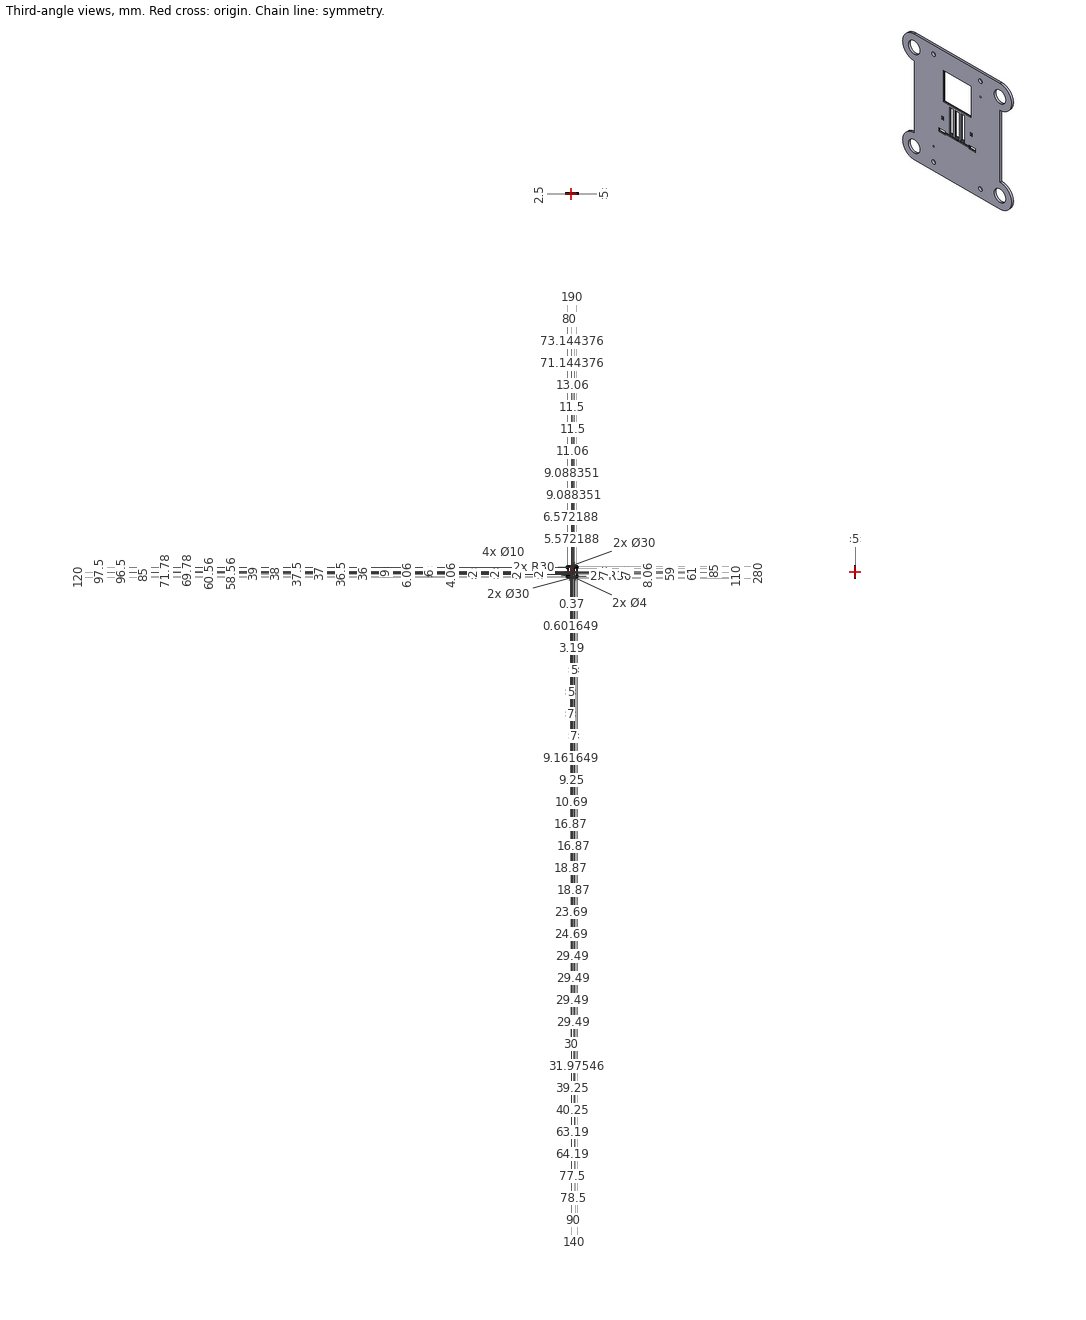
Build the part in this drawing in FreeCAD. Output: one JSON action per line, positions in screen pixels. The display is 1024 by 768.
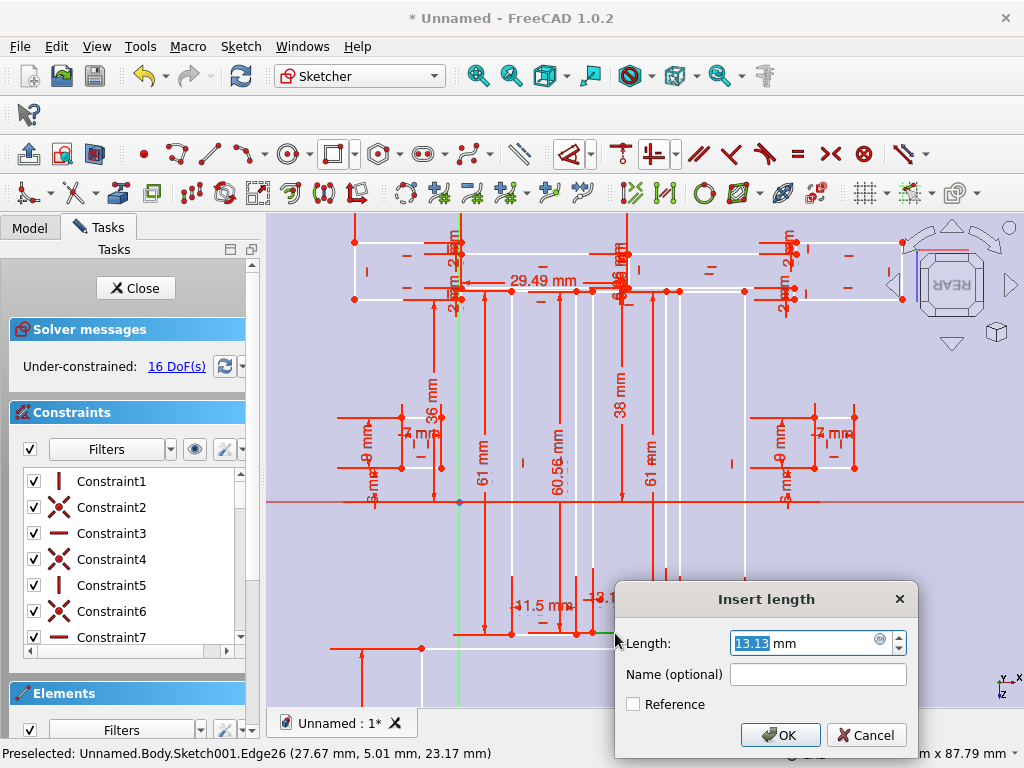
{"action": "type", "text": "13.06"}
{"action": "key", "text": "Return"}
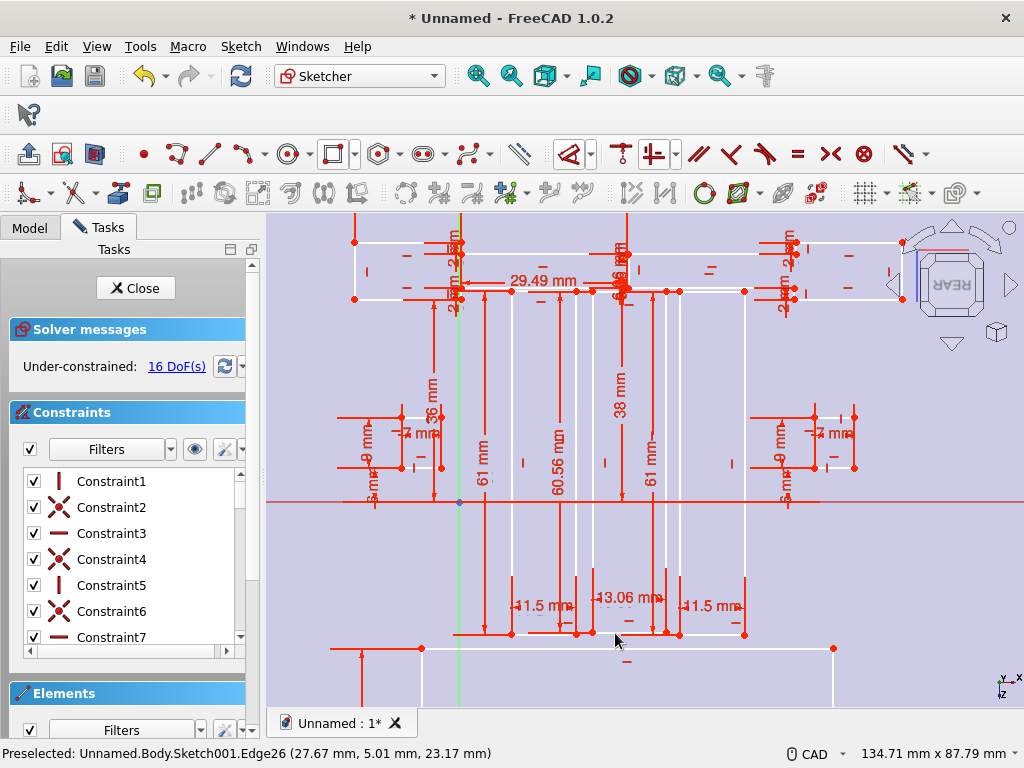
{"action": "left_click", "coordinate": [761, 288]}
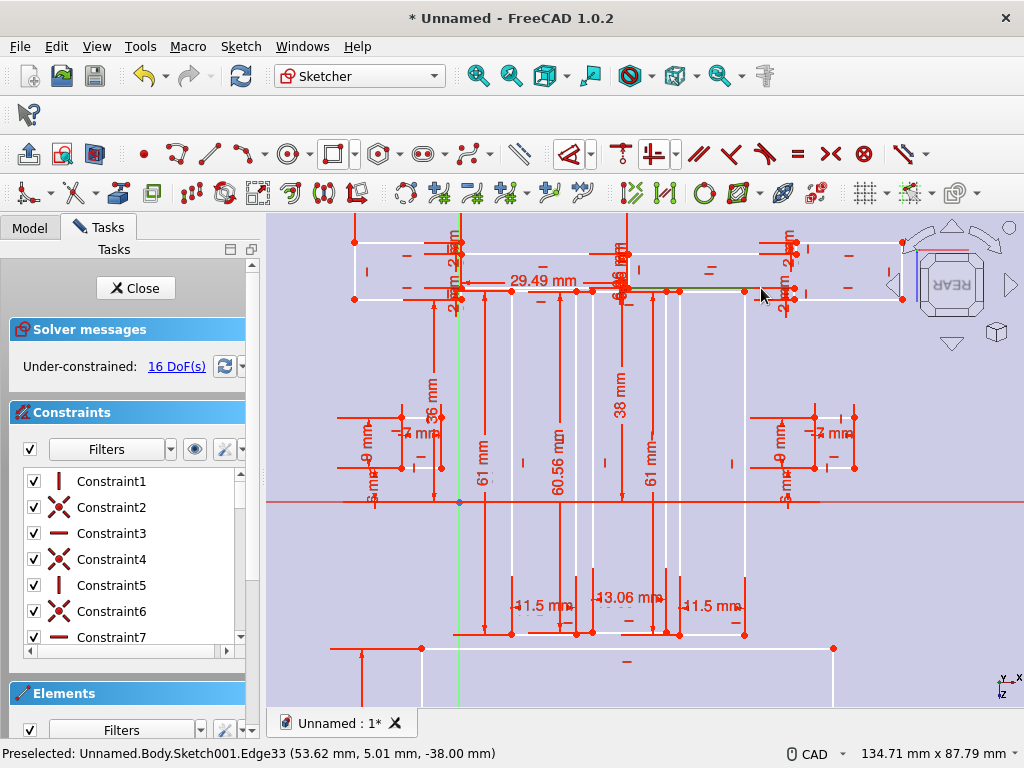
{"action": "key", "text": "l"}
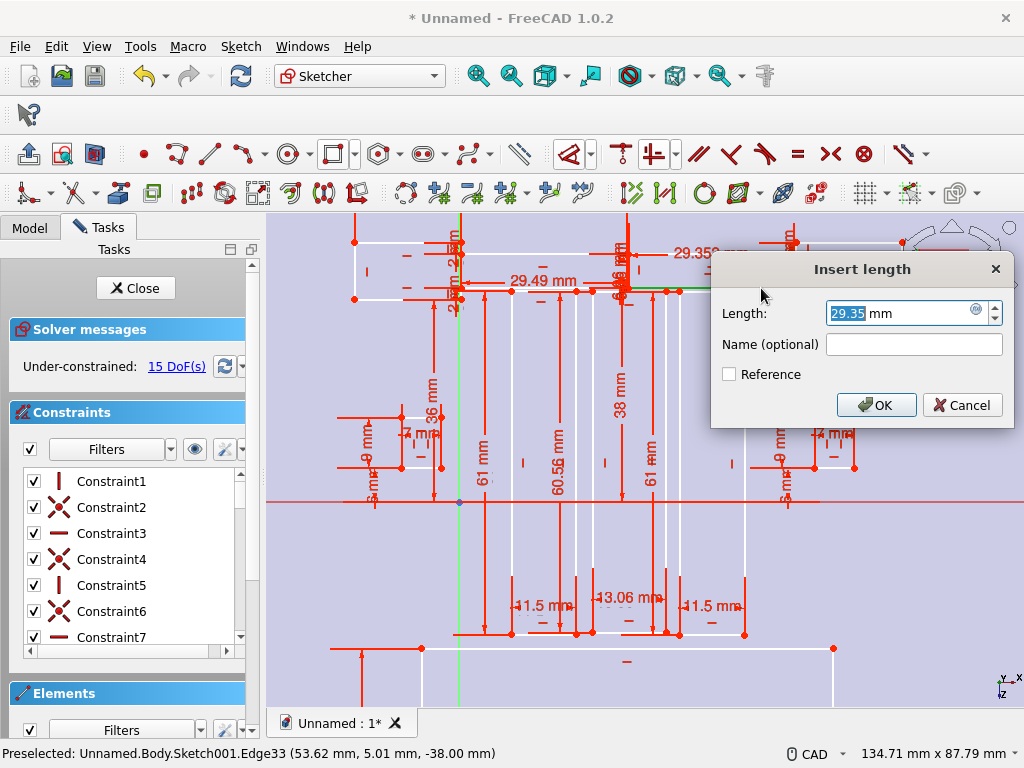
{"action": "type", "text": "29.49"}
{"action": "key", "text": "Return"}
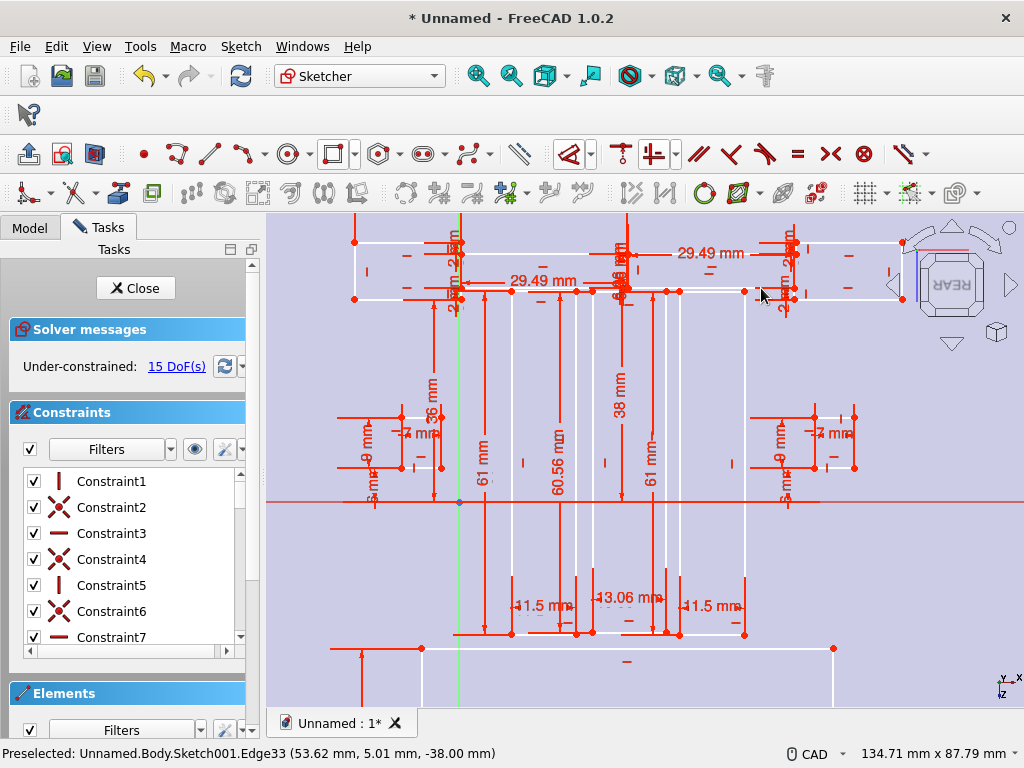
{"action": "left_click", "coordinate": [827, 300]}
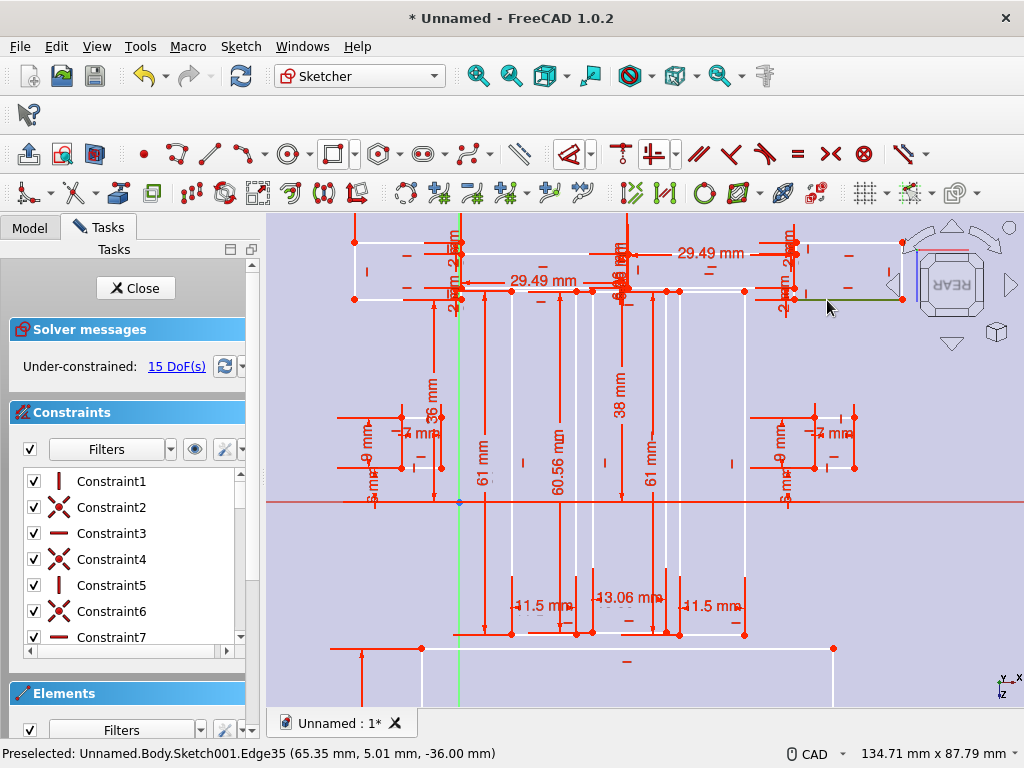
{"action": "key", "text": "l"}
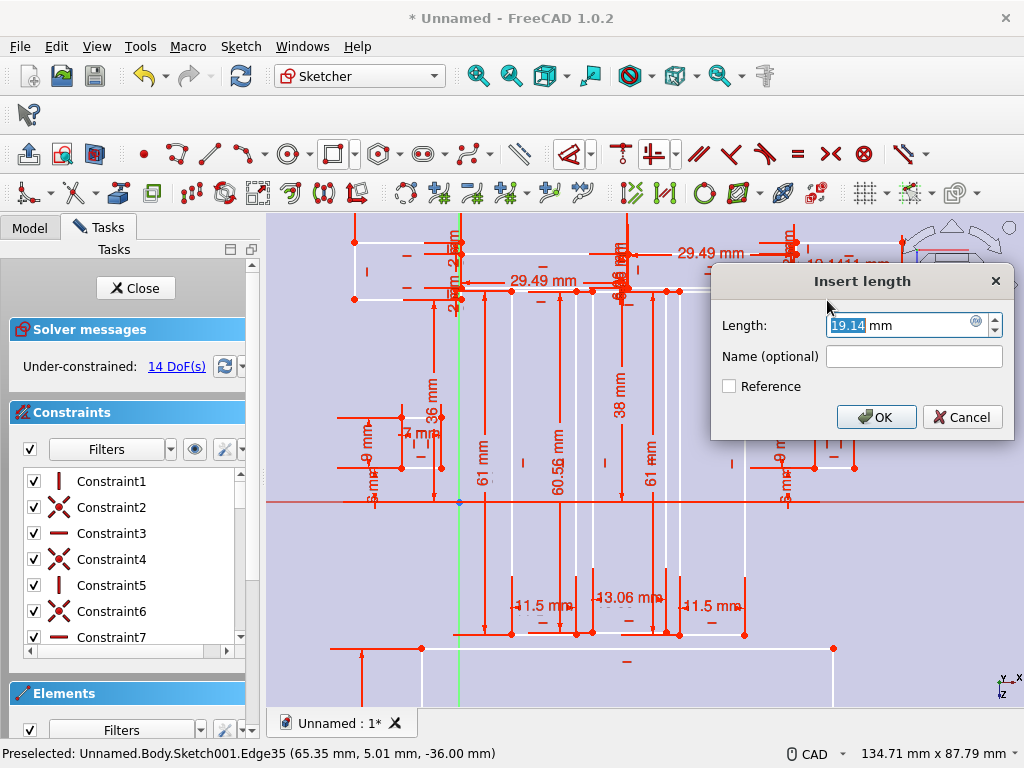
{"action": "type", "text": "18.87"}
{"action": "key", "text": "Return"}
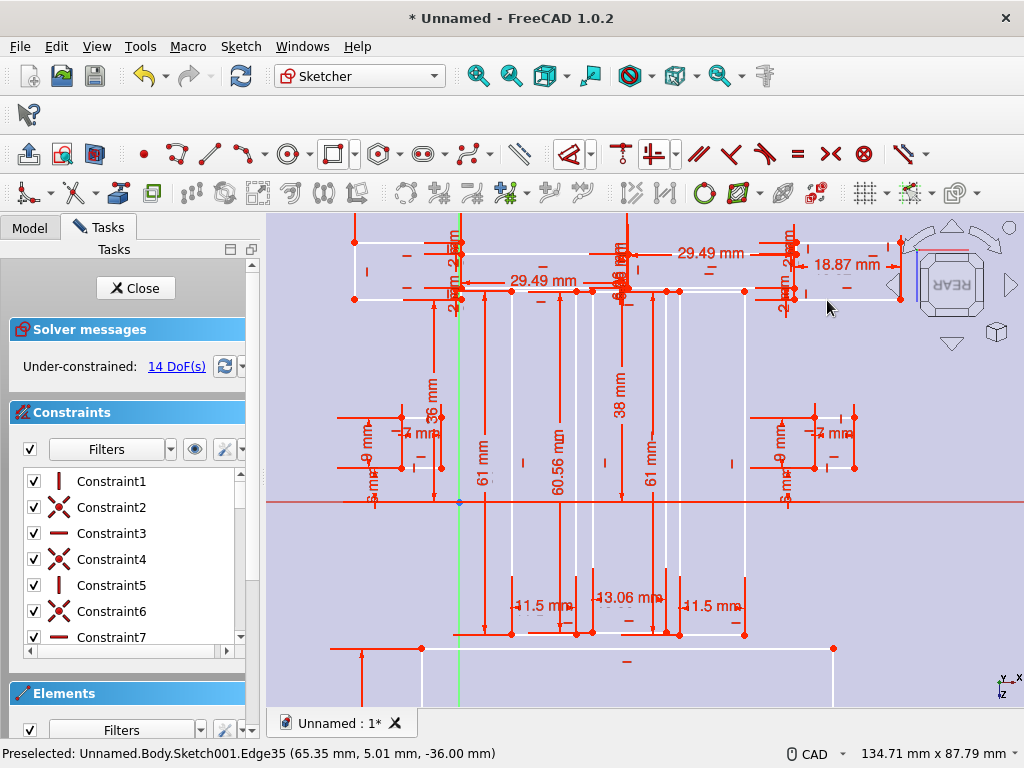
{"action": "left_click", "coordinate": [827, 243]}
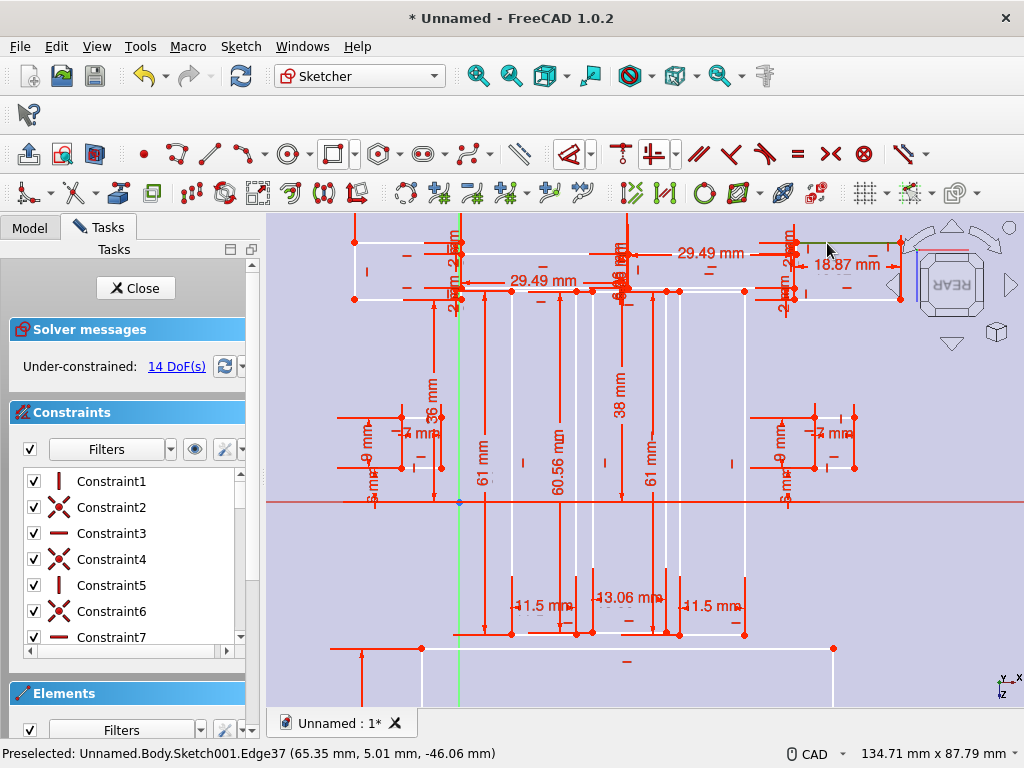
{"action": "left_click", "coordinate": [590, 154]}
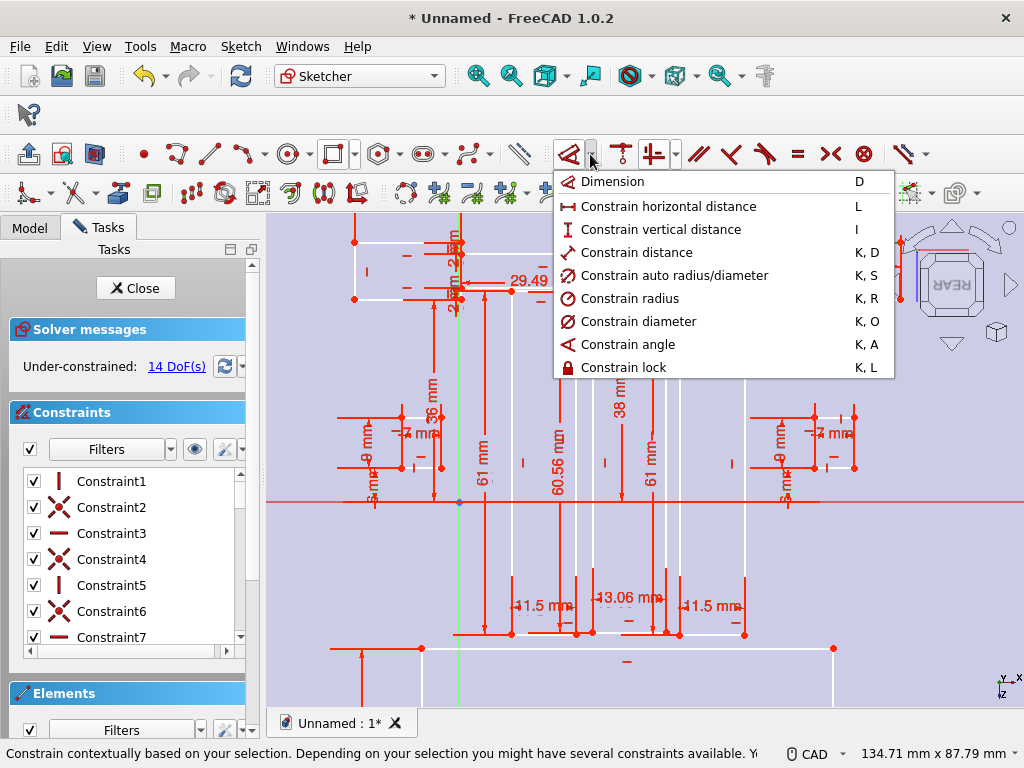
{"action": "left_click", "coordinate": [724, 206]}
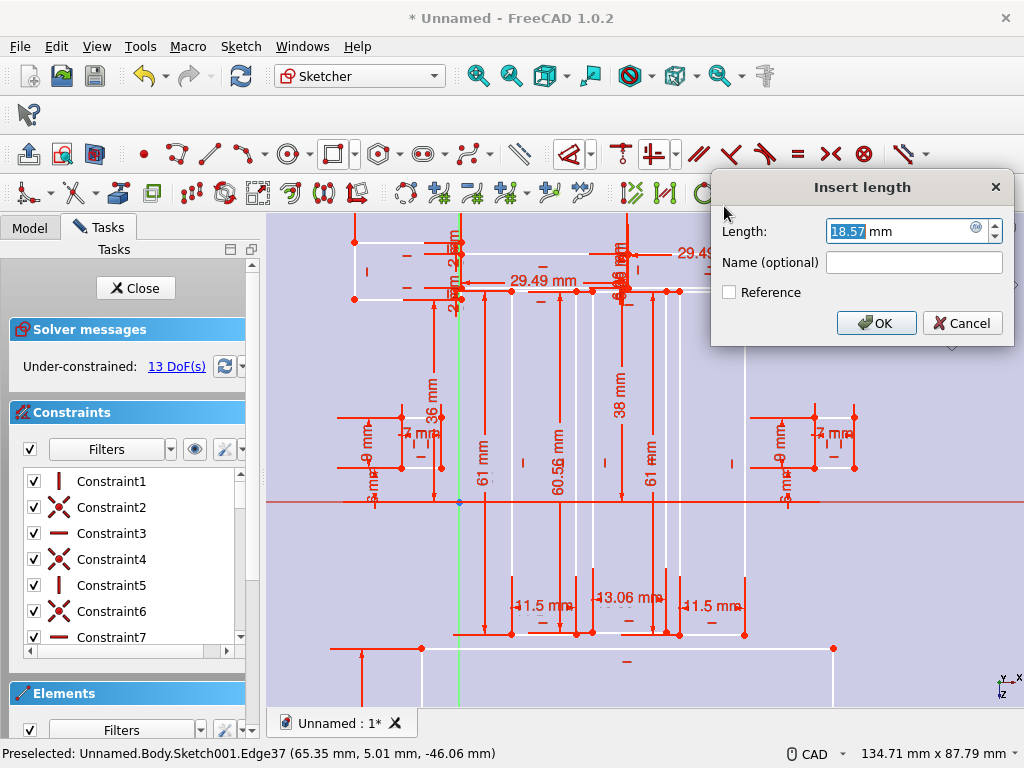
{"action": "type", "text": "18.87"}
{"action": "key", "text": "Return"}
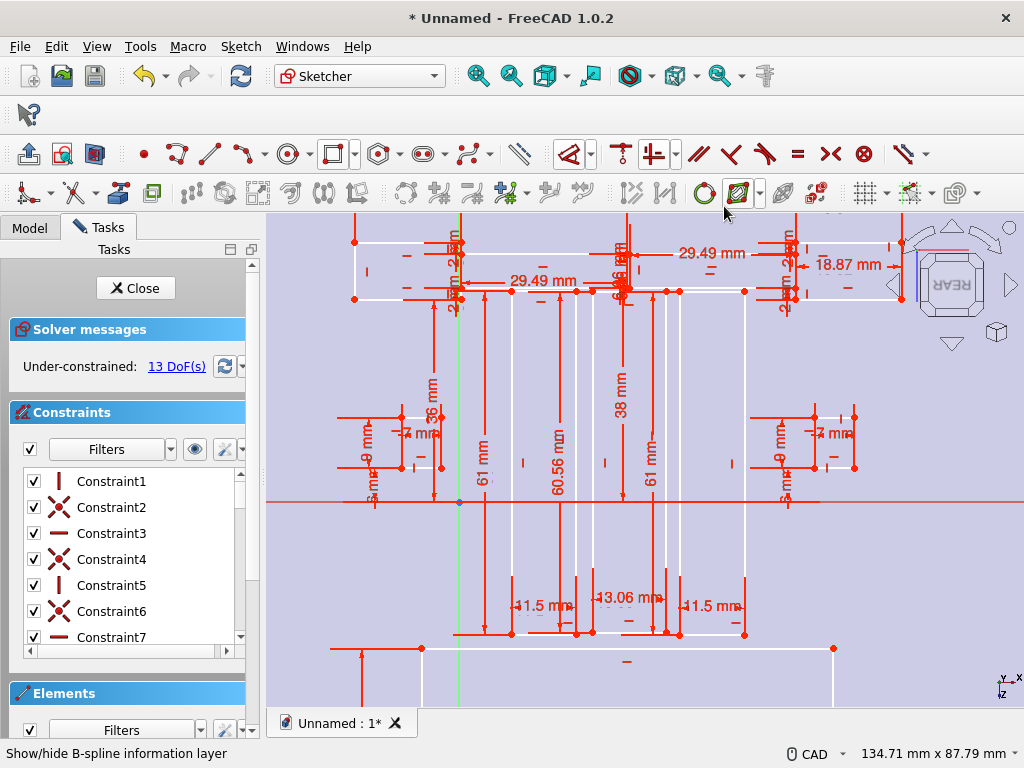
{"action": "scroll", "coordinate": [461, 300], "scroll_direction": "up", "scroll_amount": 15}